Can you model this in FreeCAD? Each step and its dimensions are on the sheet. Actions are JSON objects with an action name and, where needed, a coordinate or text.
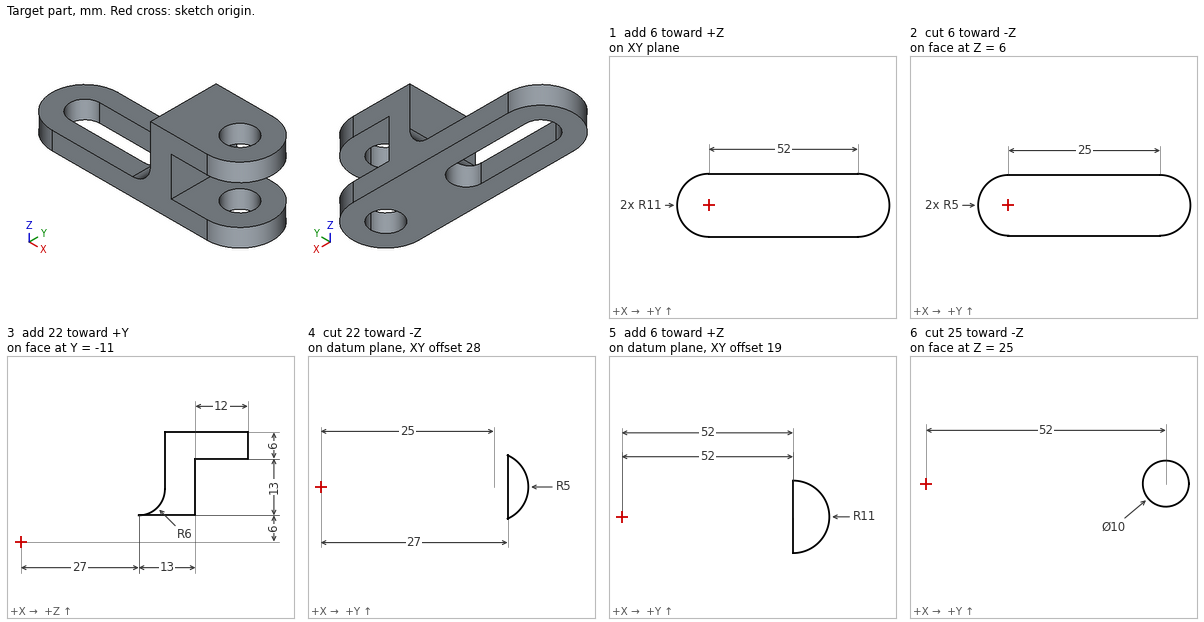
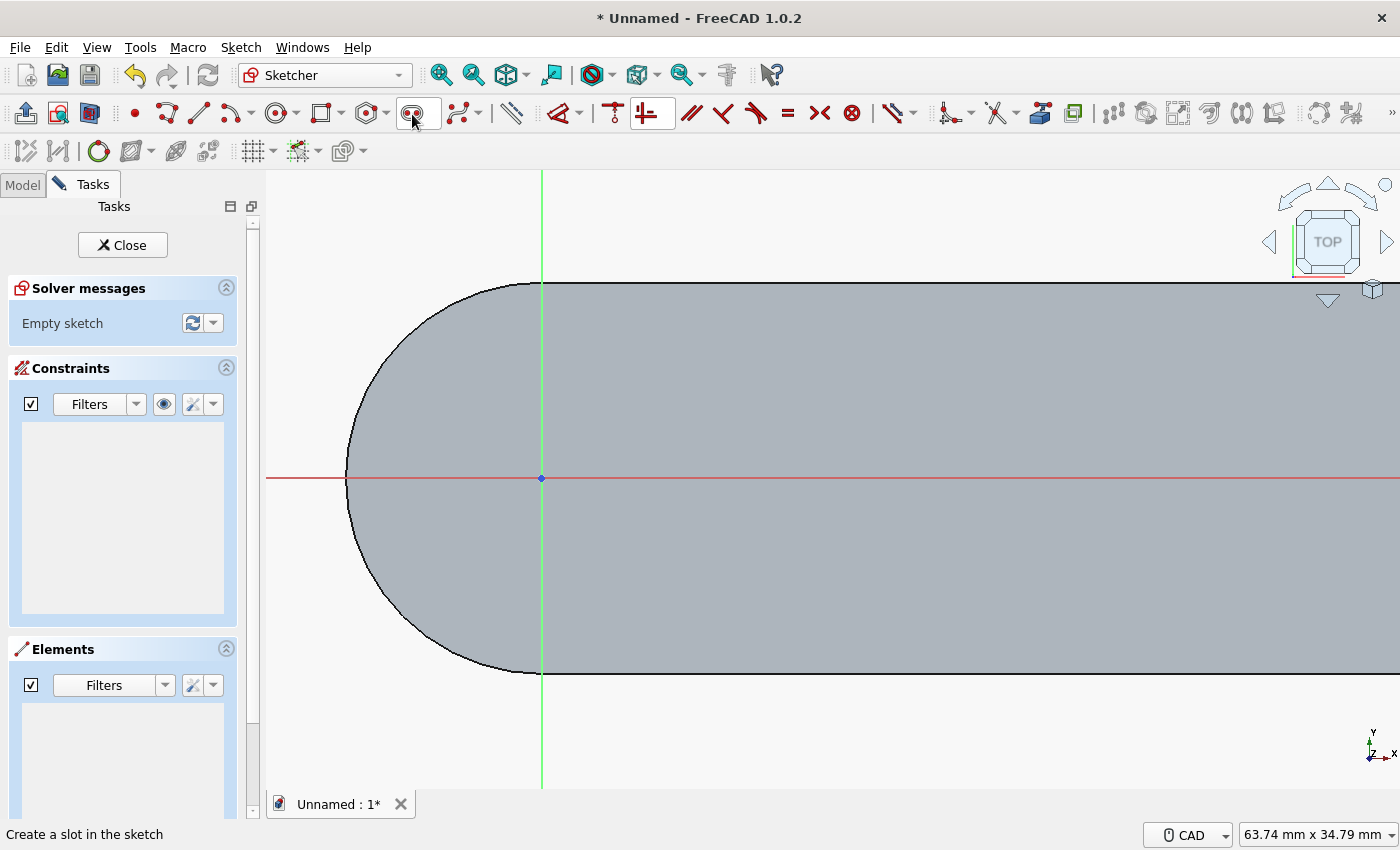
{"action": "left_click", "coordinate": [542, 478]}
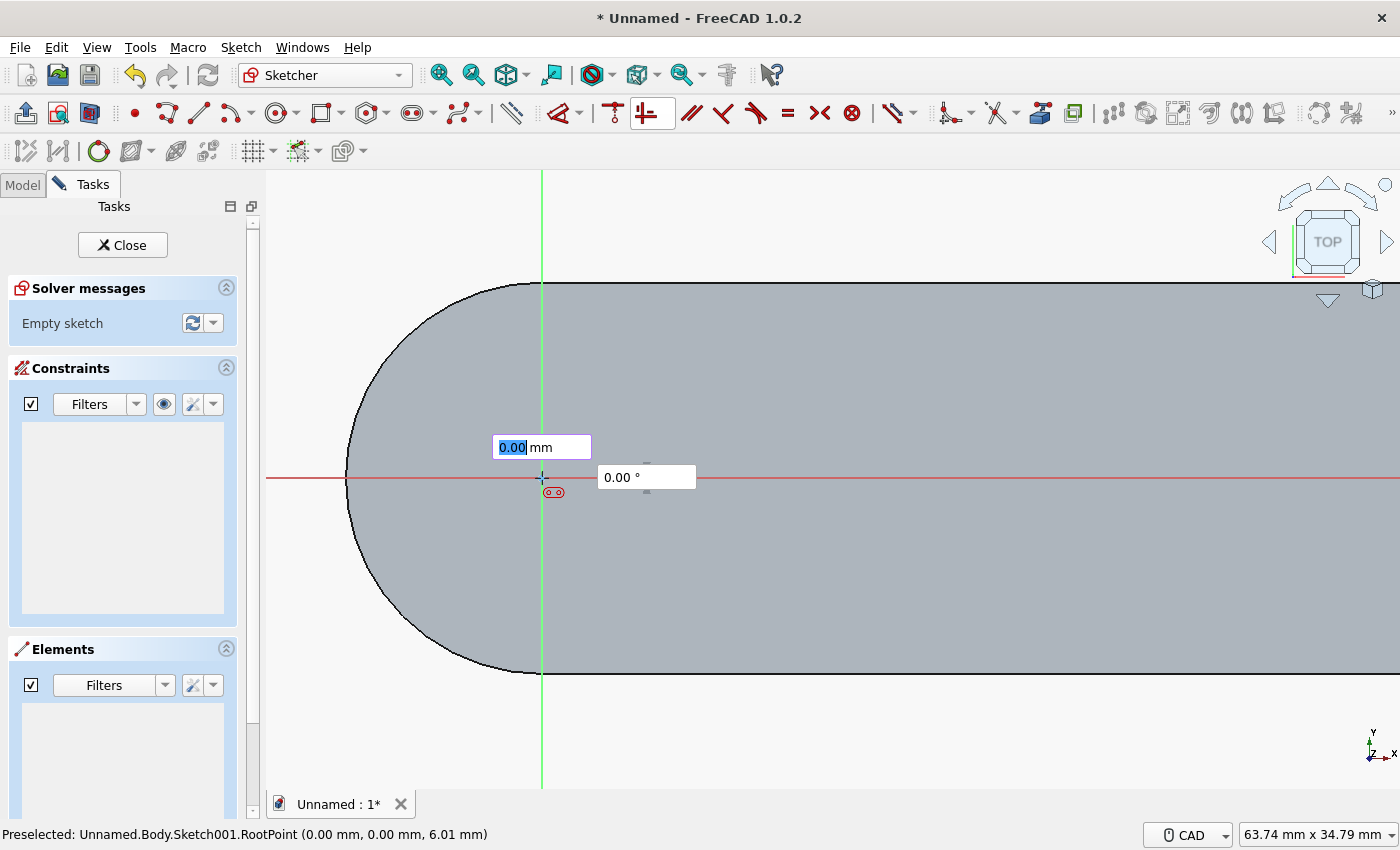
{"action": "left_click", "coordinate": [986, 469]}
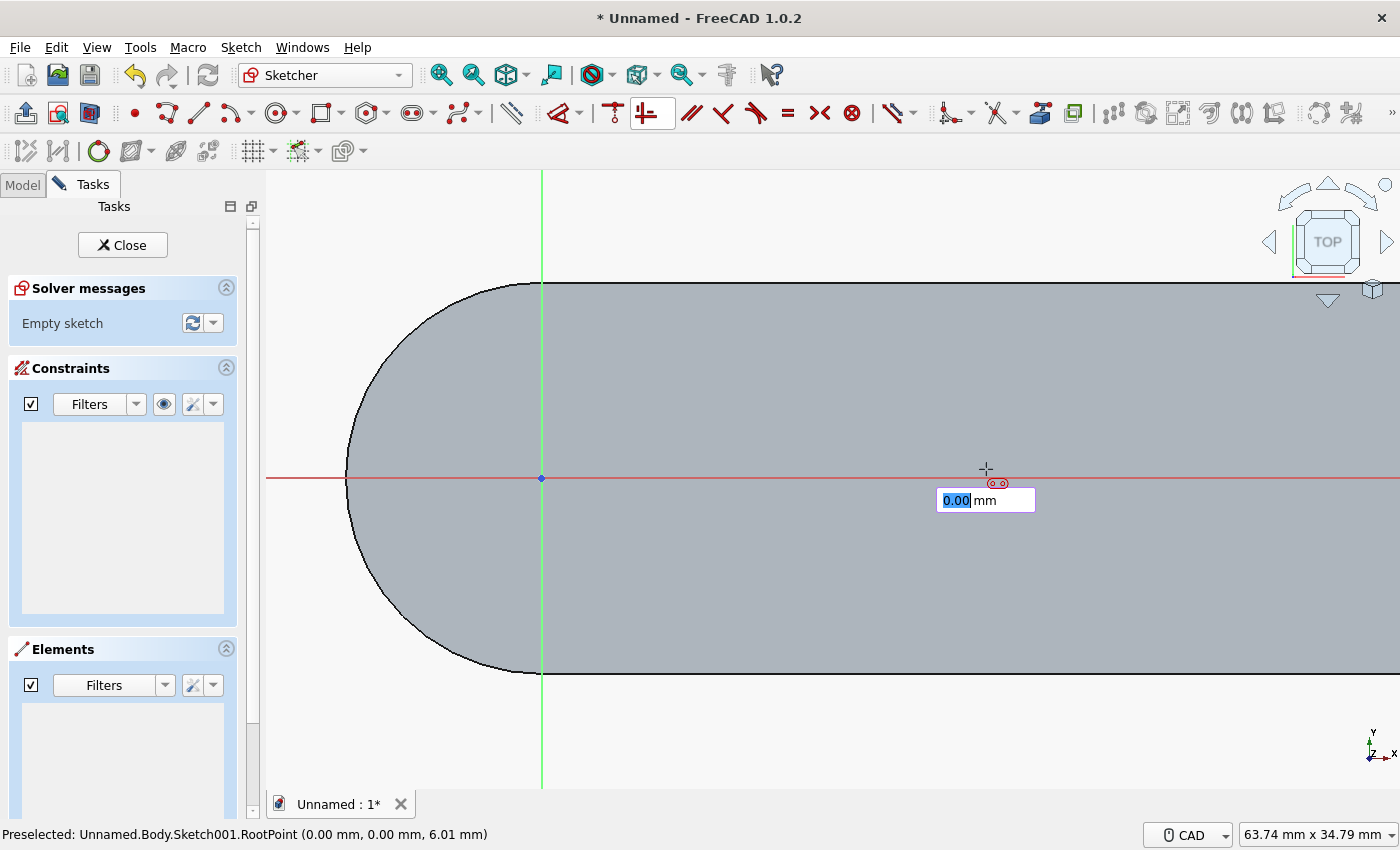
{"action": "left_click", "coordinate": [764, 389]}
{"action": "key", "text": "Escape"}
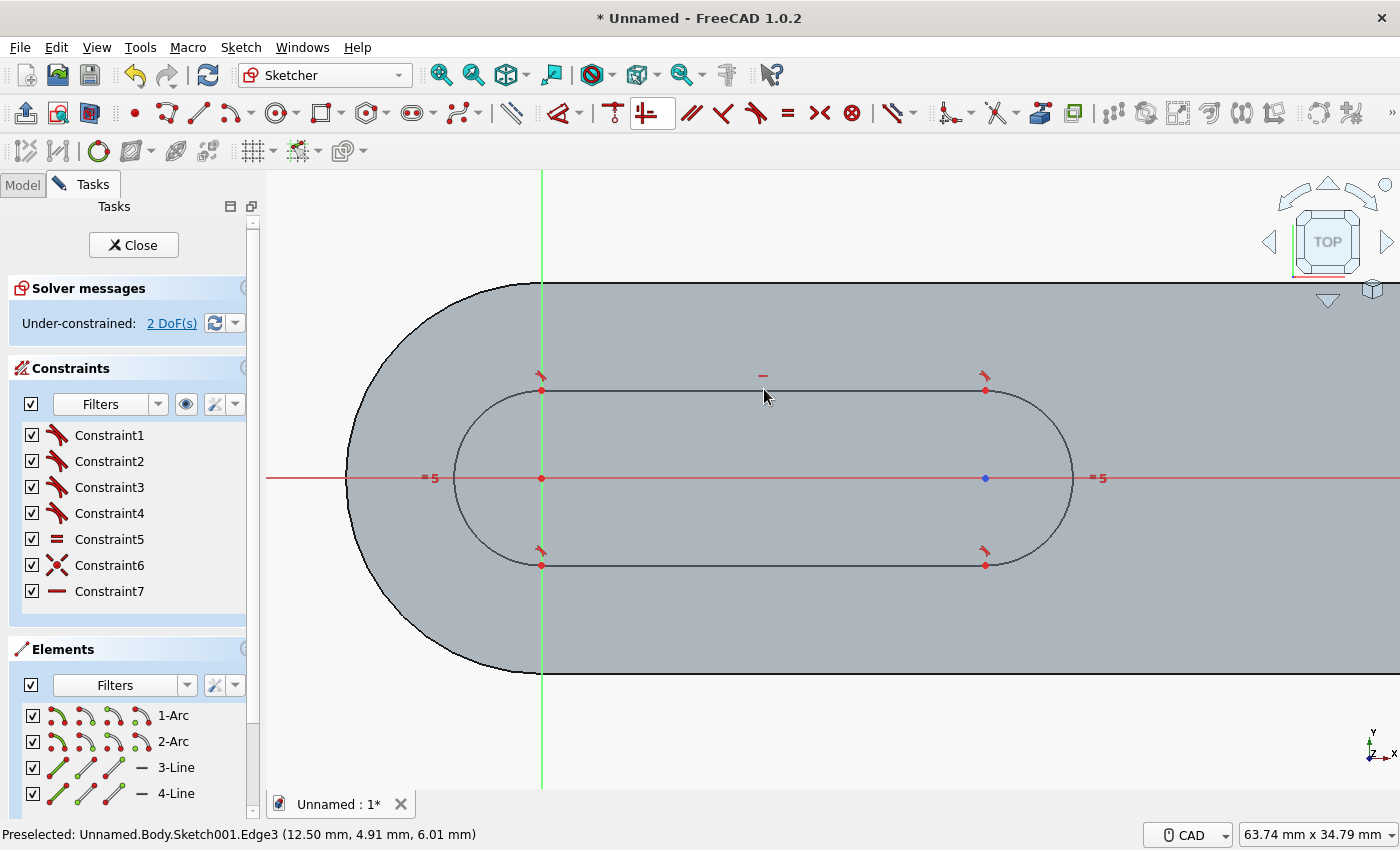
{"action": "left_click", "coordinate": [558, 114]}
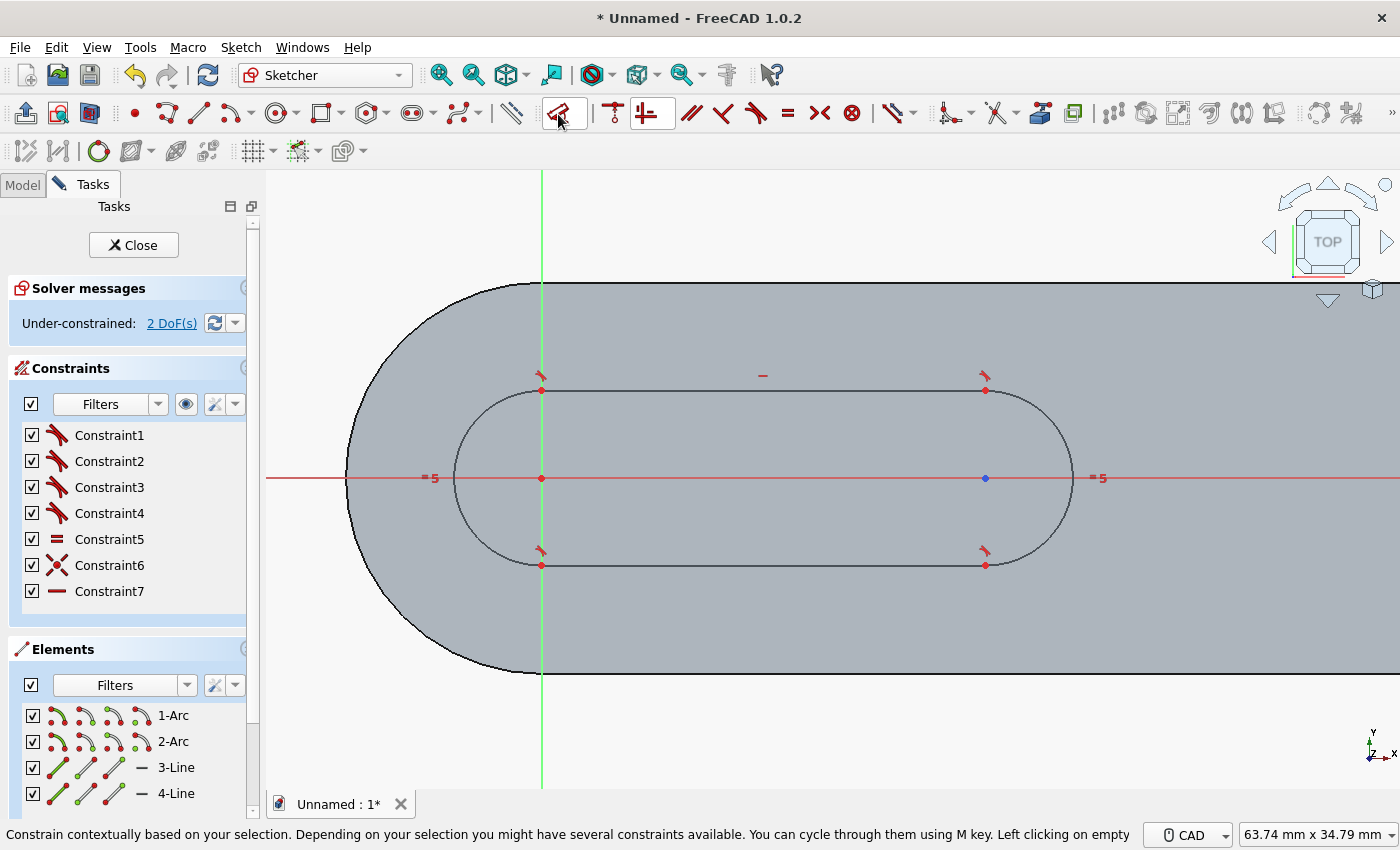
{"action": "left_click", "coordinate": [471, 427]}
{"action": "left_click", "coordinate": [445, 408]}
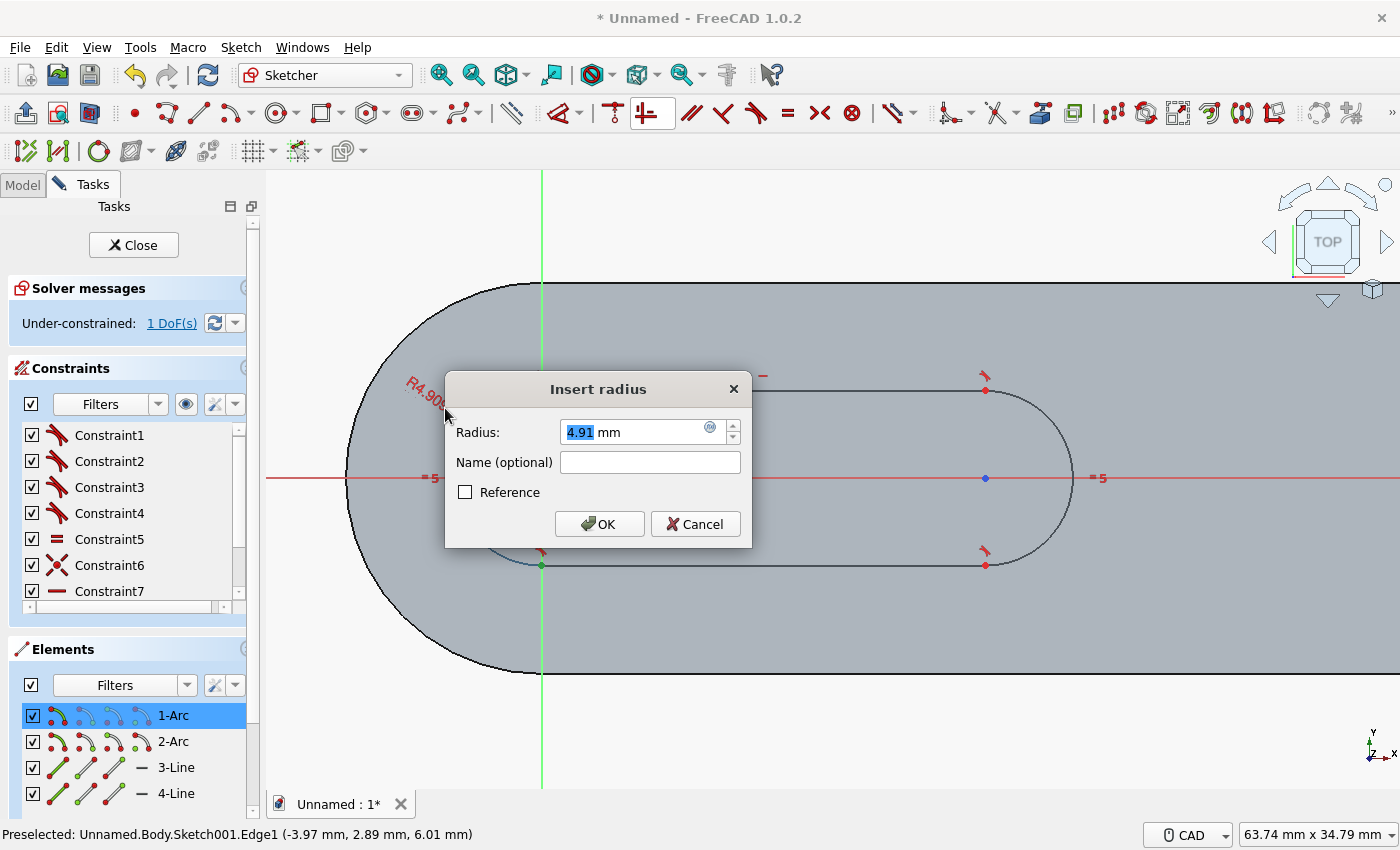
{"action": "type", "text": "5"}
{"action": "key", "text": "Return"}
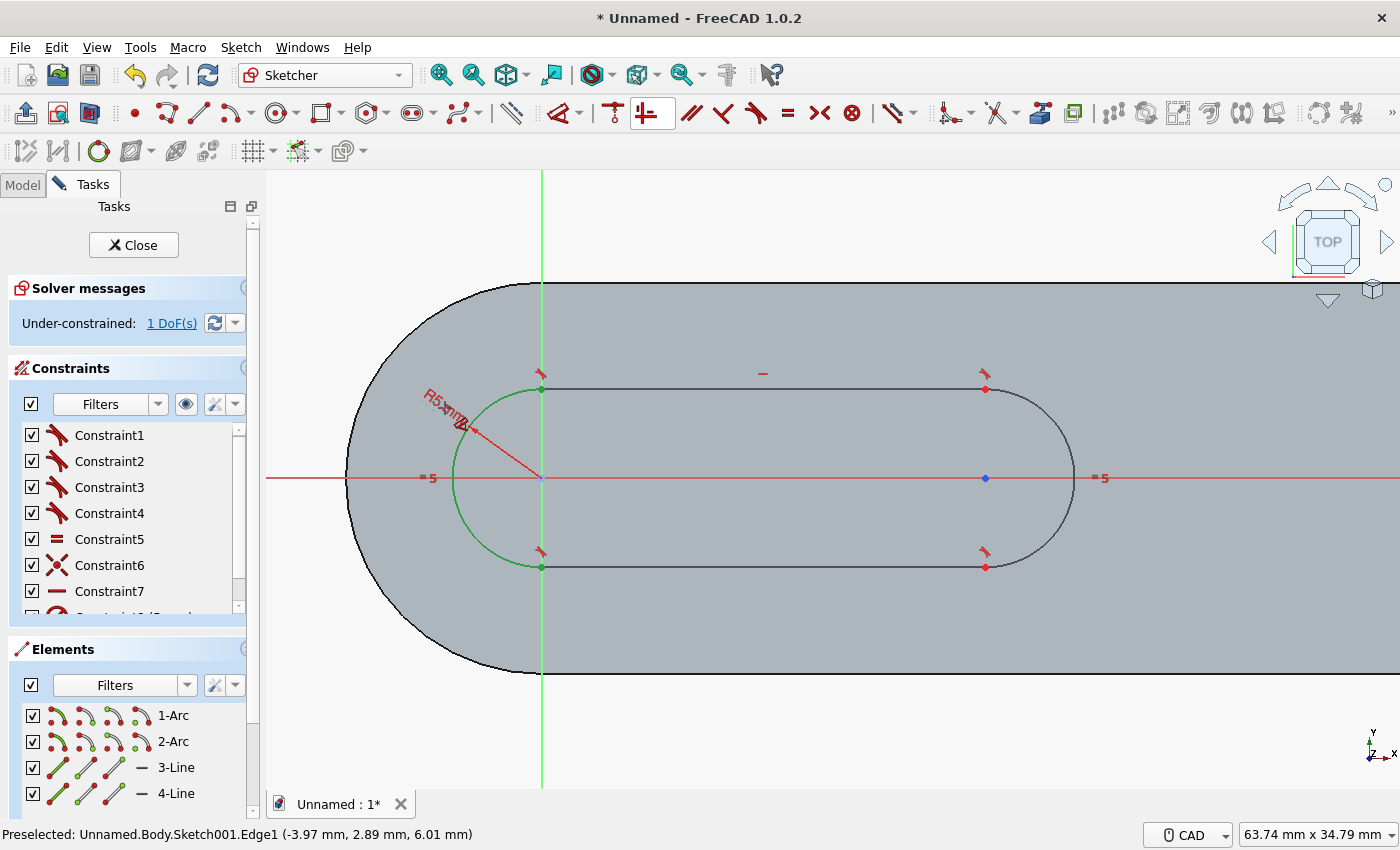
{"action": "left_click", "coordinate": [675, 389]}
{"action": "left_click", "coordinate": [764, 355]}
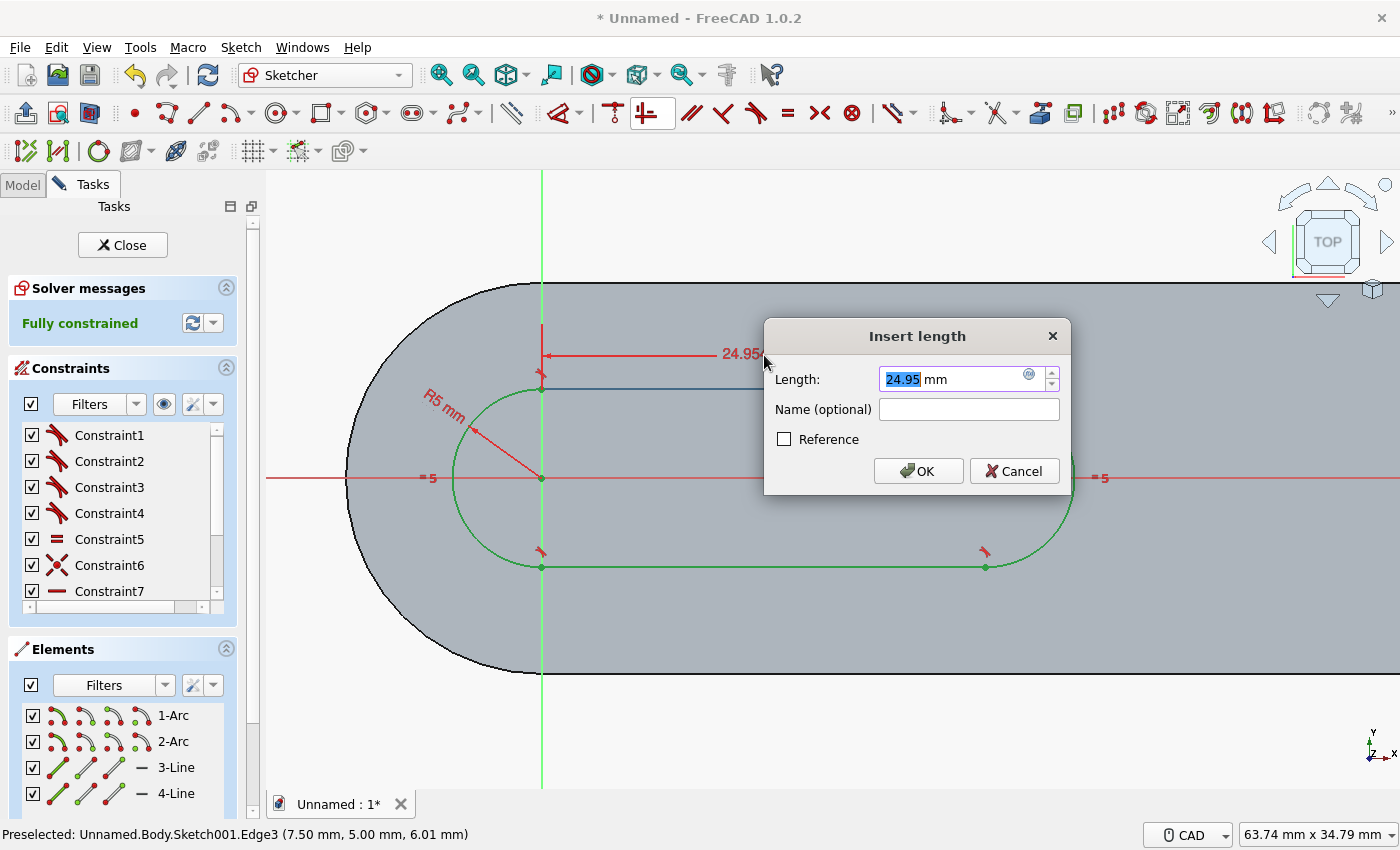
{"action": "type", "text": "25"}
{"action": "key", "text": "Return"}
{"action": "key", "text": "Escape"}